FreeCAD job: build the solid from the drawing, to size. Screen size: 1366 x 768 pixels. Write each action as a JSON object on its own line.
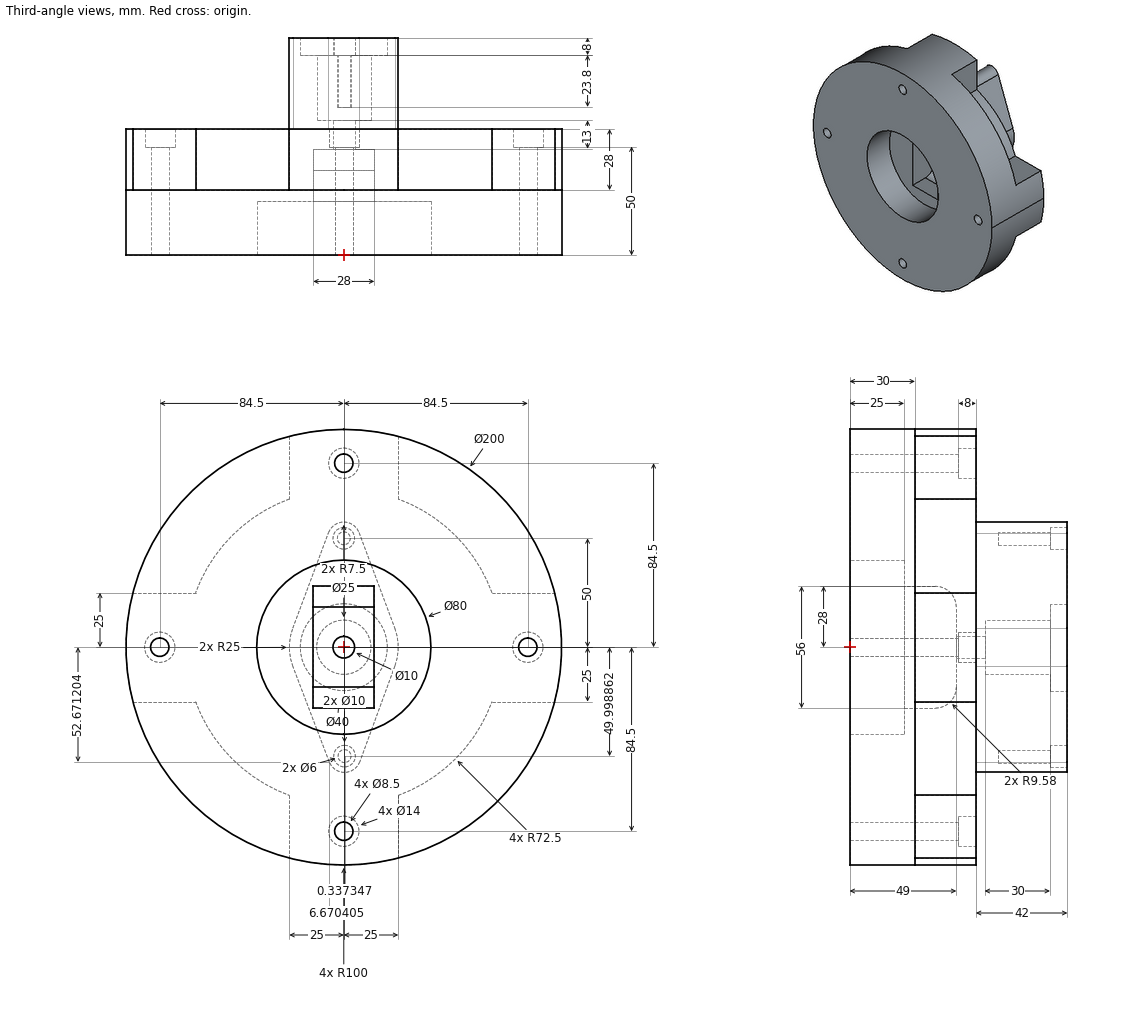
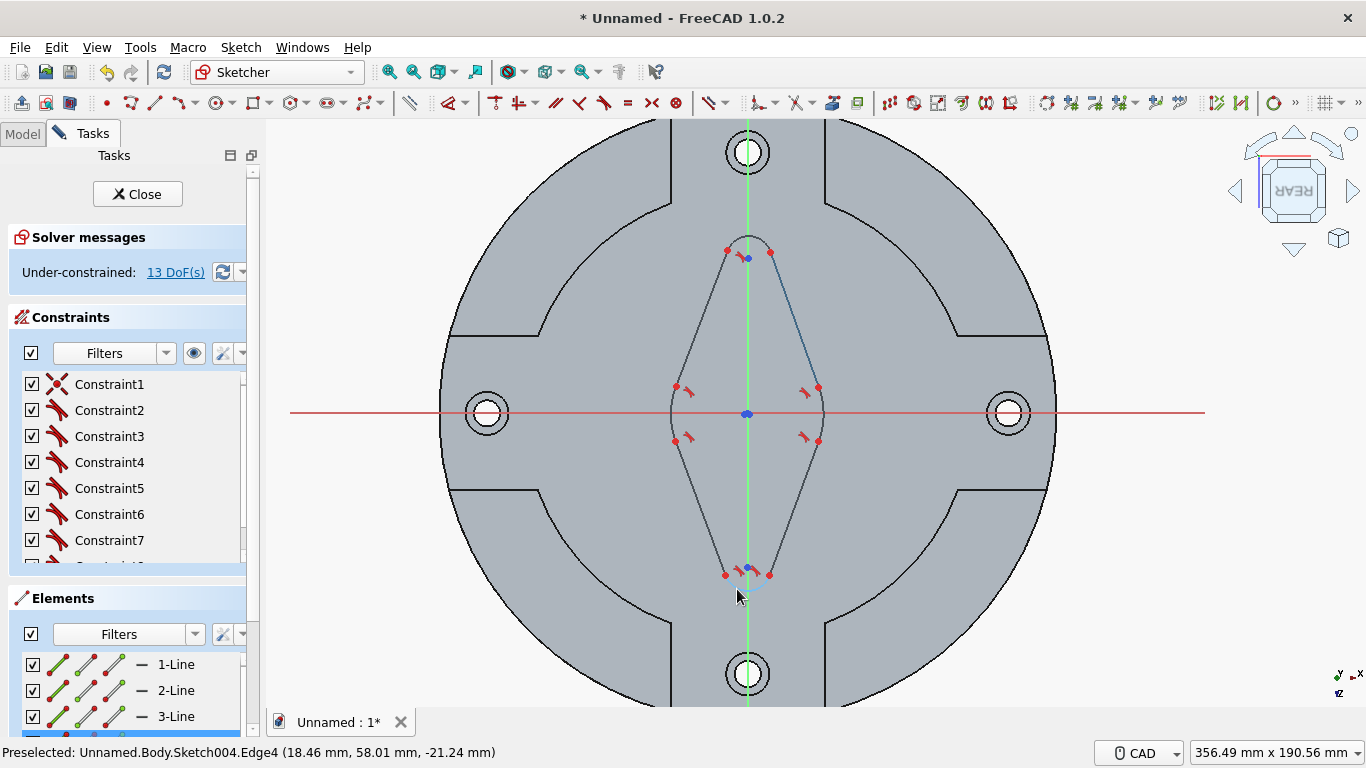
{"action": "left_click", "coordinate": [761, 239]}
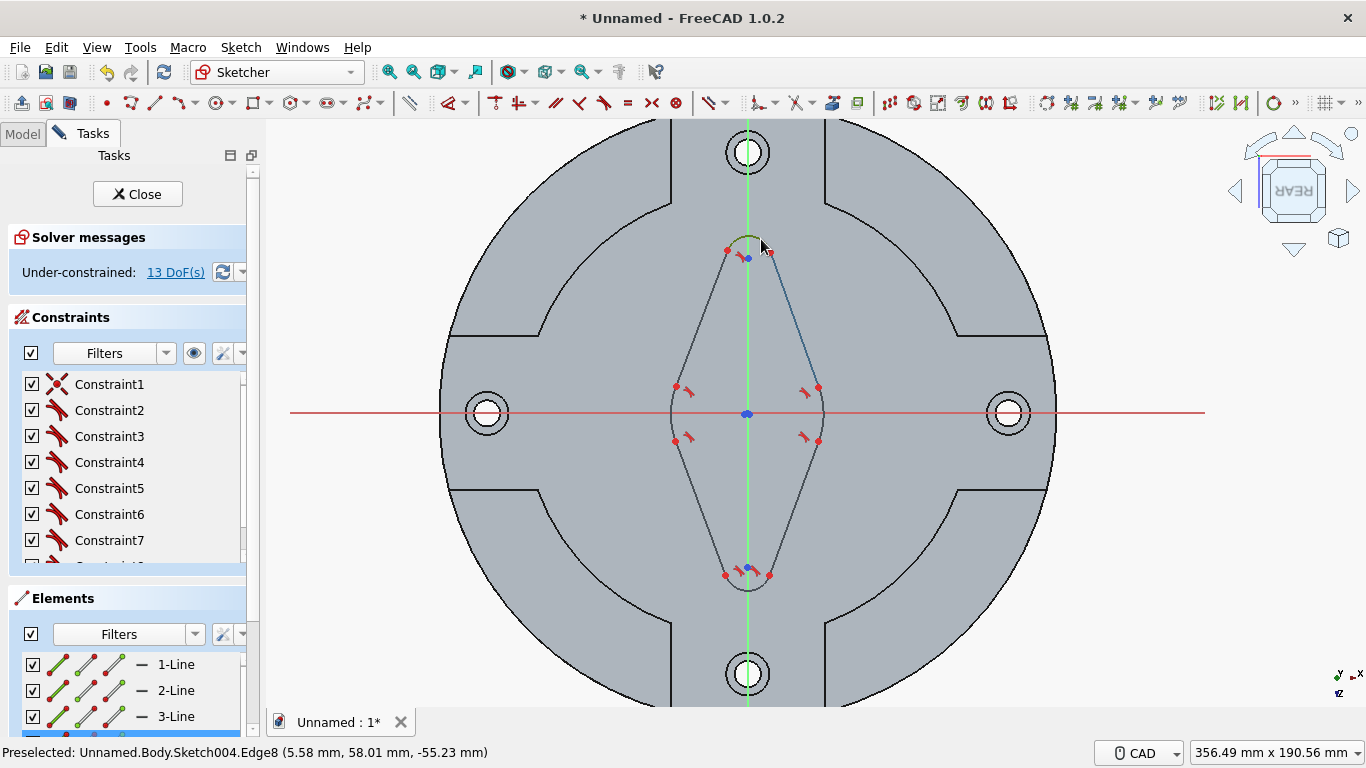
{"action": "key", "text": "t"}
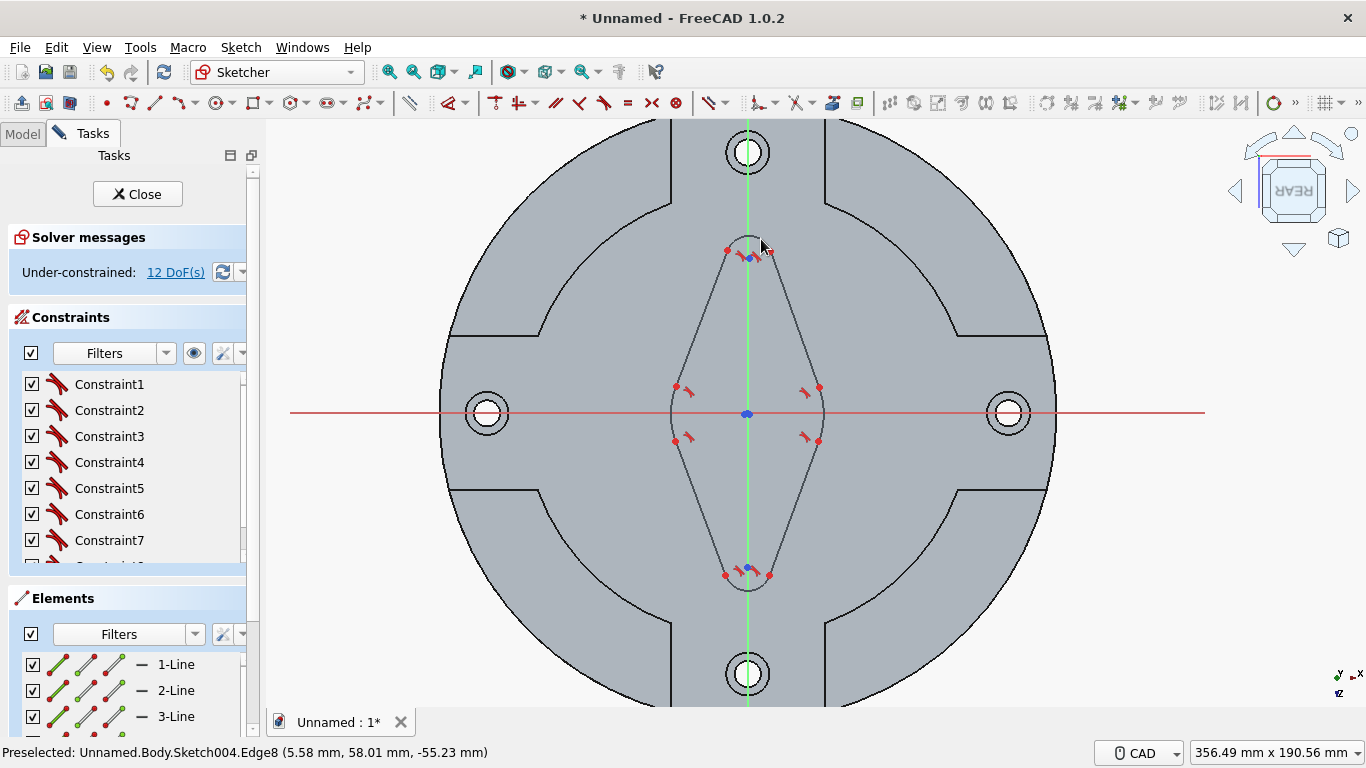
{"action": "scroll", "coordinate": [672, 403], "scroll_direction": "up", "scroll_amount": 2}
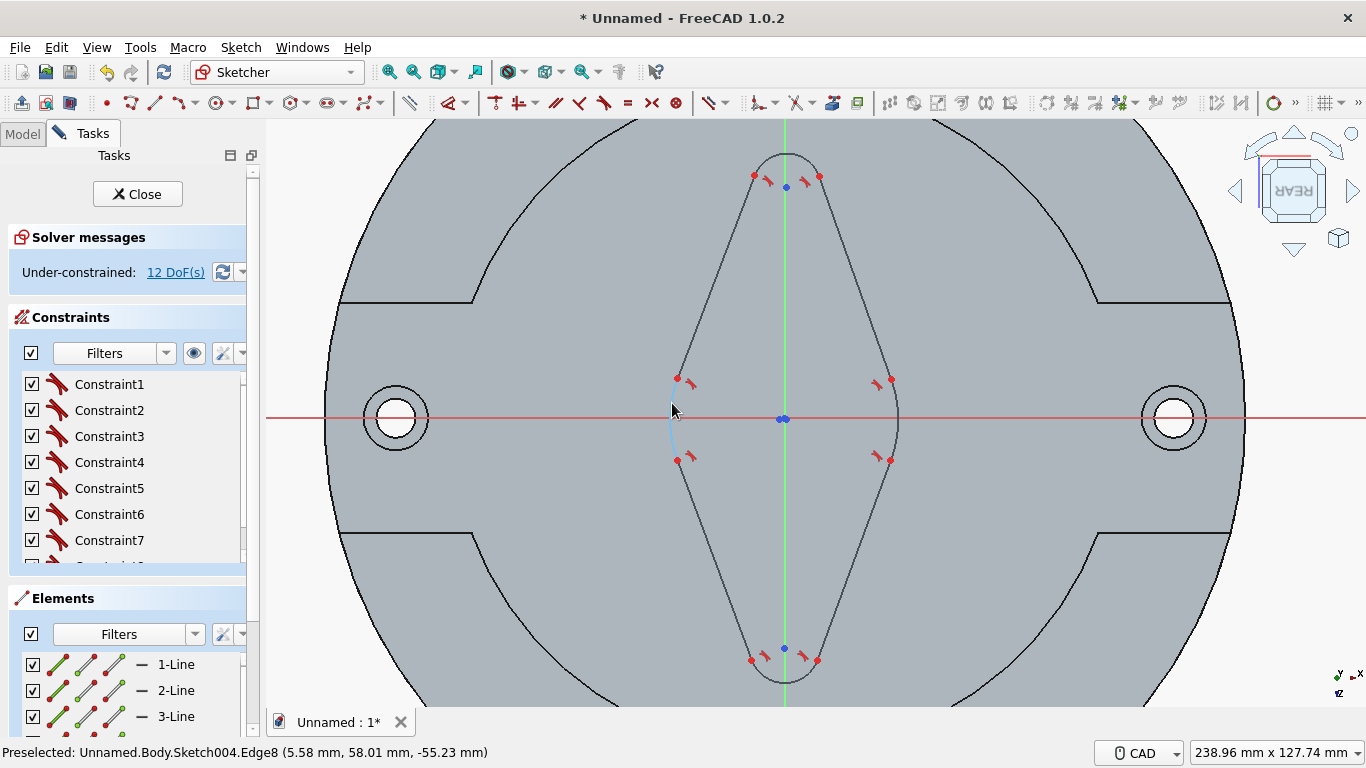
{"action": "left_click", "coordinate": [671, 403]}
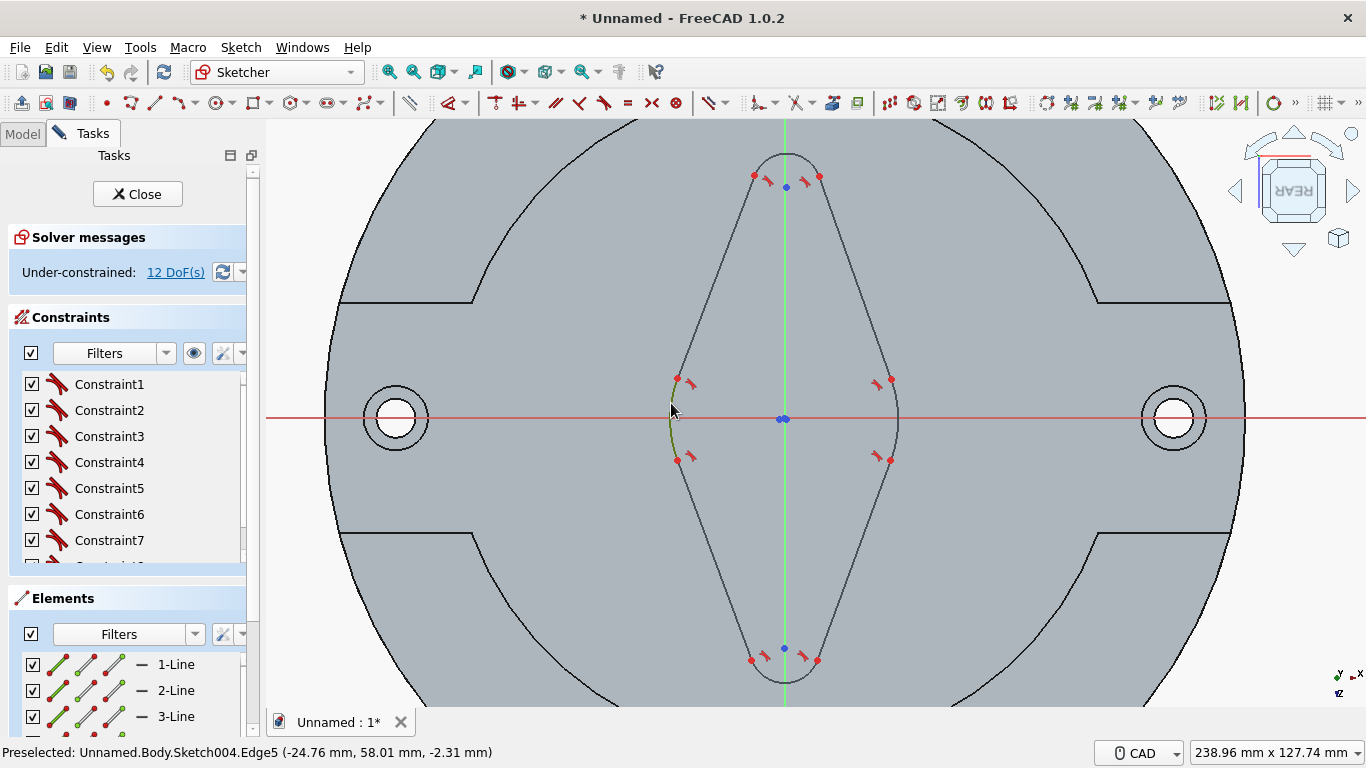
{"action": "left_click", "coordinate": [897, 436]}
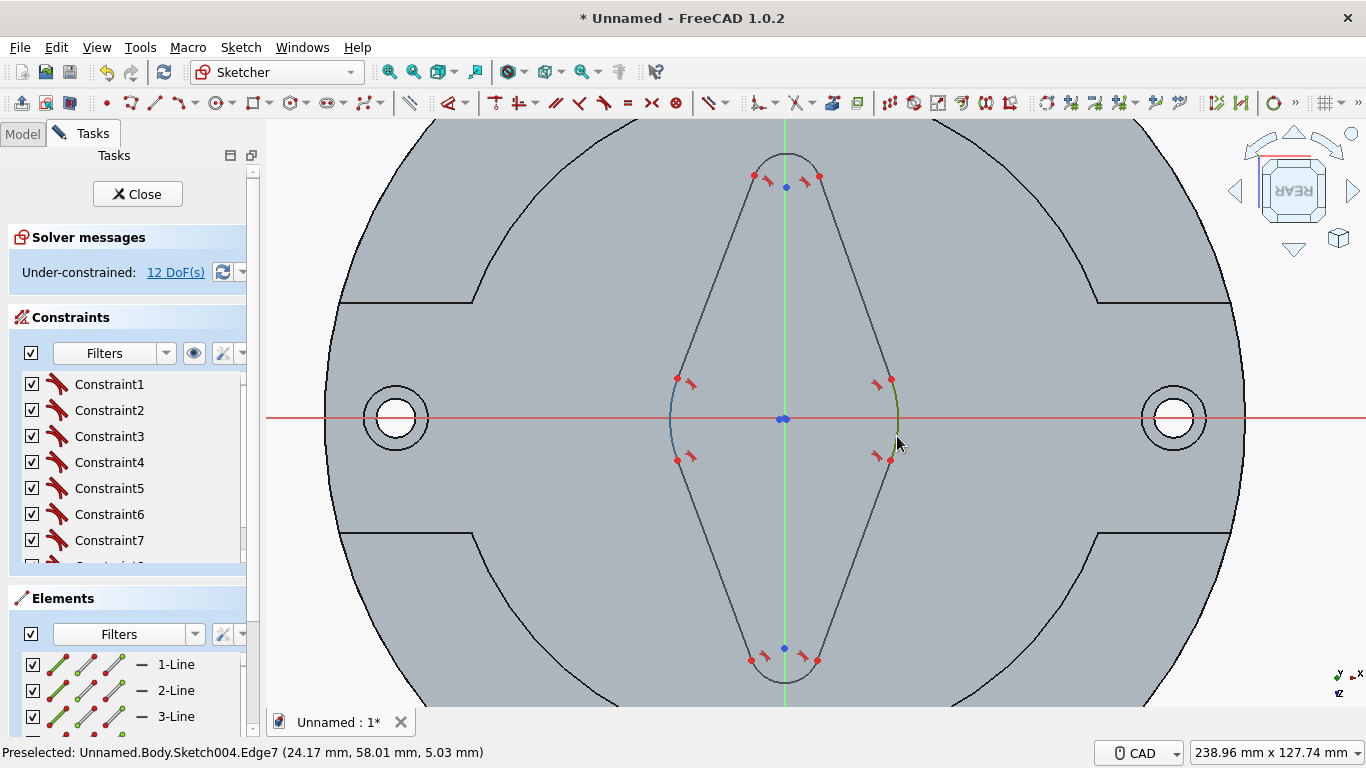
{"action": "left_click", "coordinate": [496, 104]}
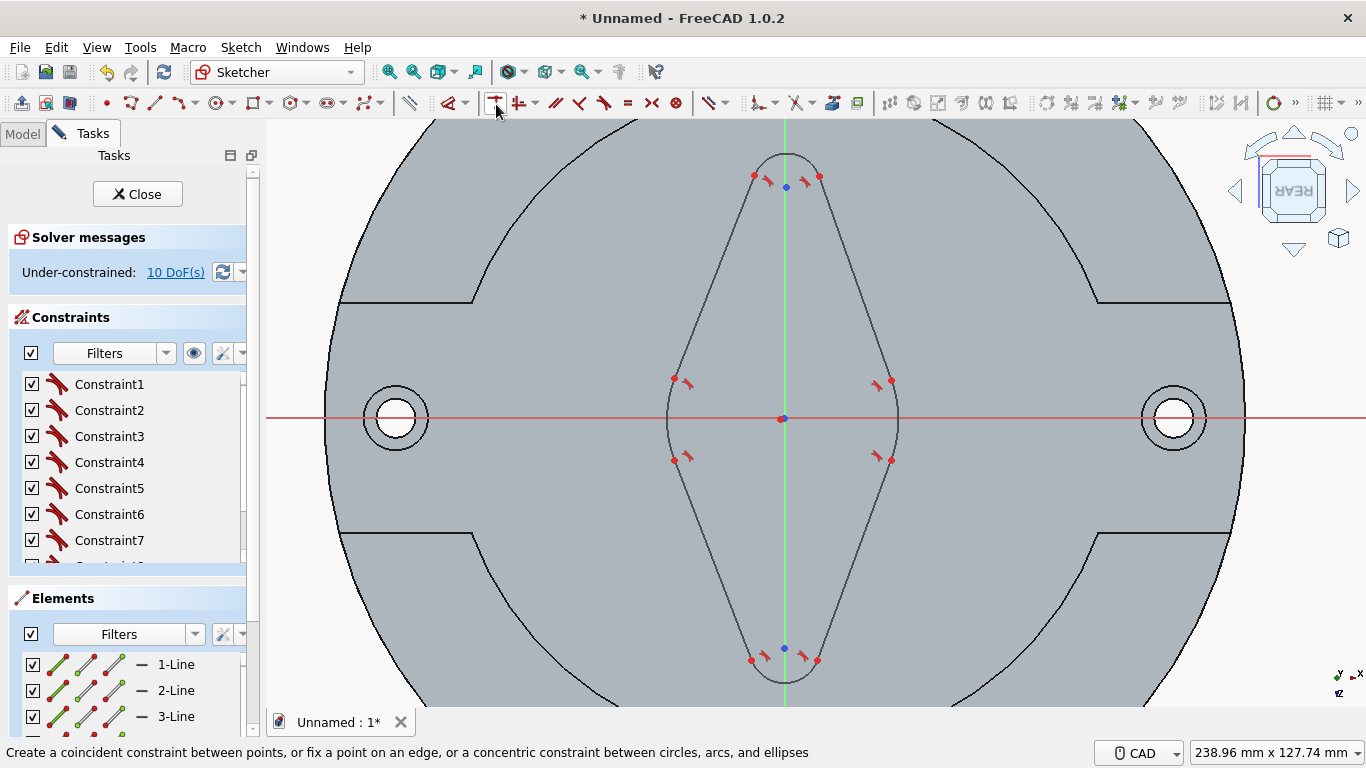
{"action": "left_click_drag", "start_coordinate": [770, 408], "coordinate": [795, 430]}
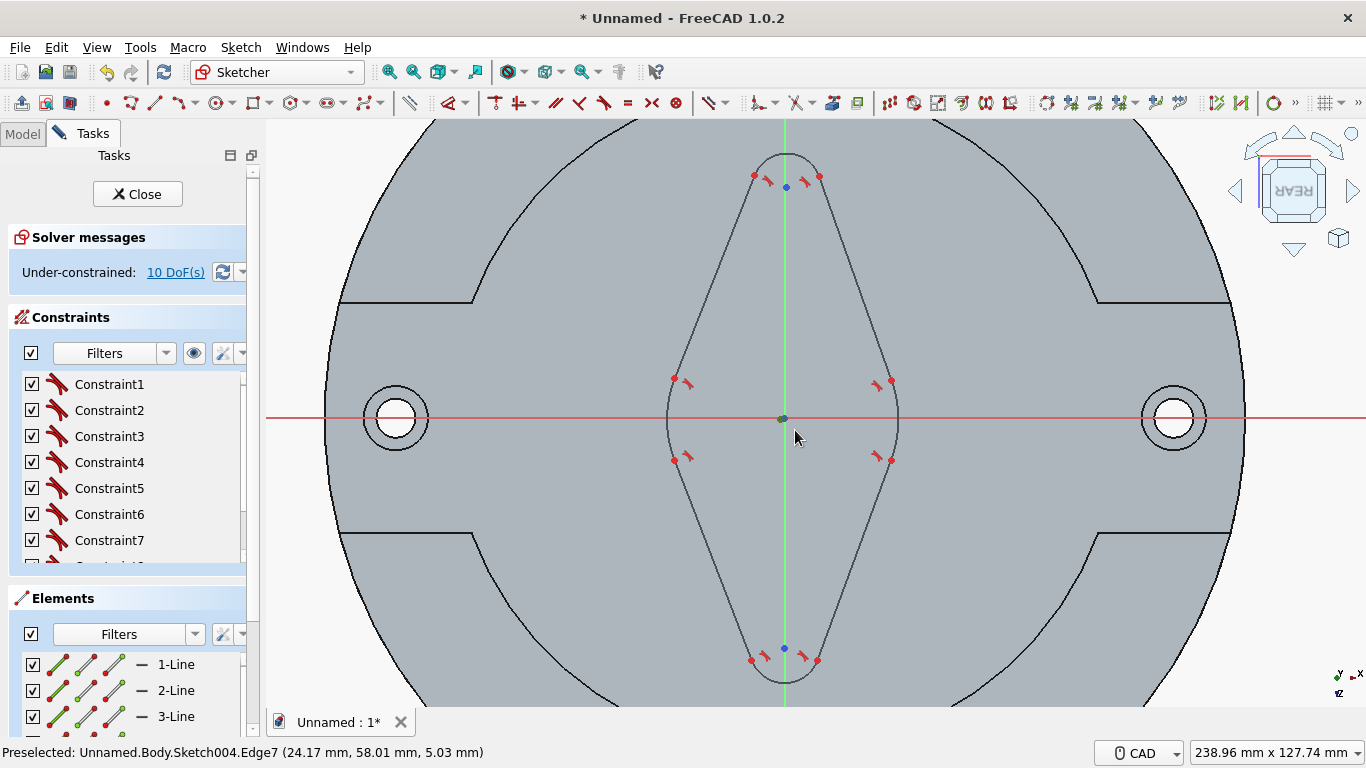
{"action": "key", "text": "c"}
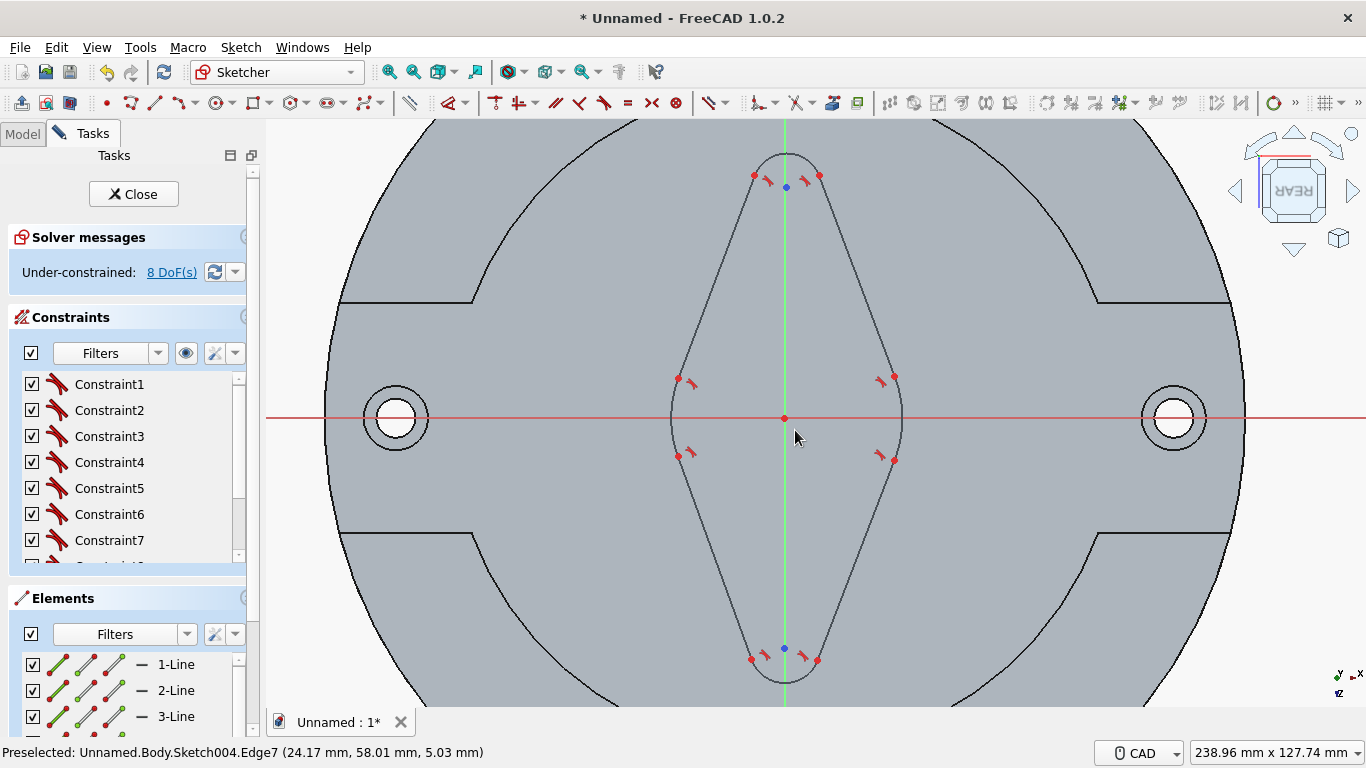
{"action": "left_click", "coordinate": [672, 401]}